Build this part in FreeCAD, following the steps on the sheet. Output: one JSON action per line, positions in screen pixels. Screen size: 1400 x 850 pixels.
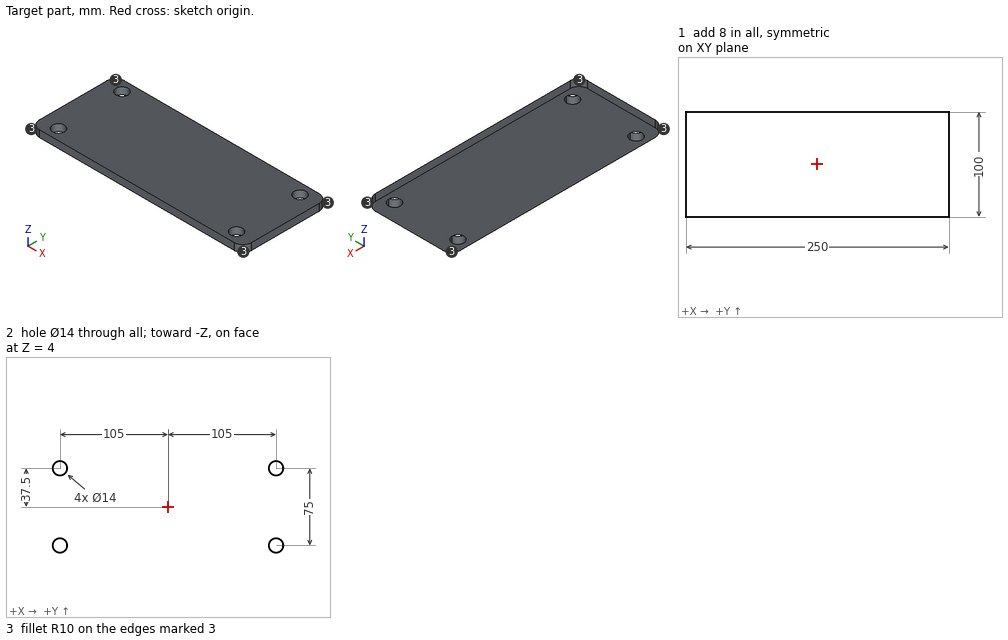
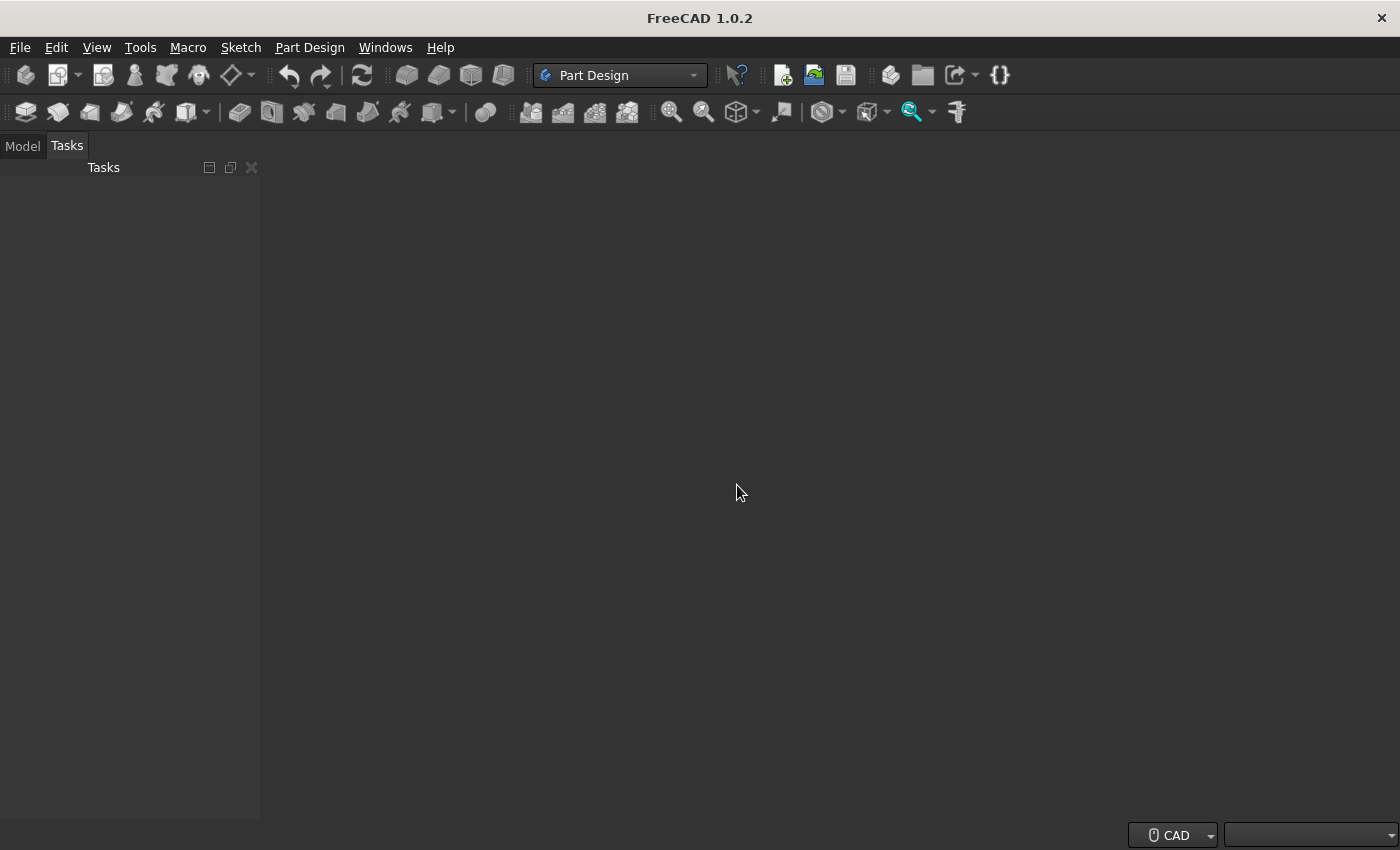
{"action": "left_click", "coordinate": [782, 76]}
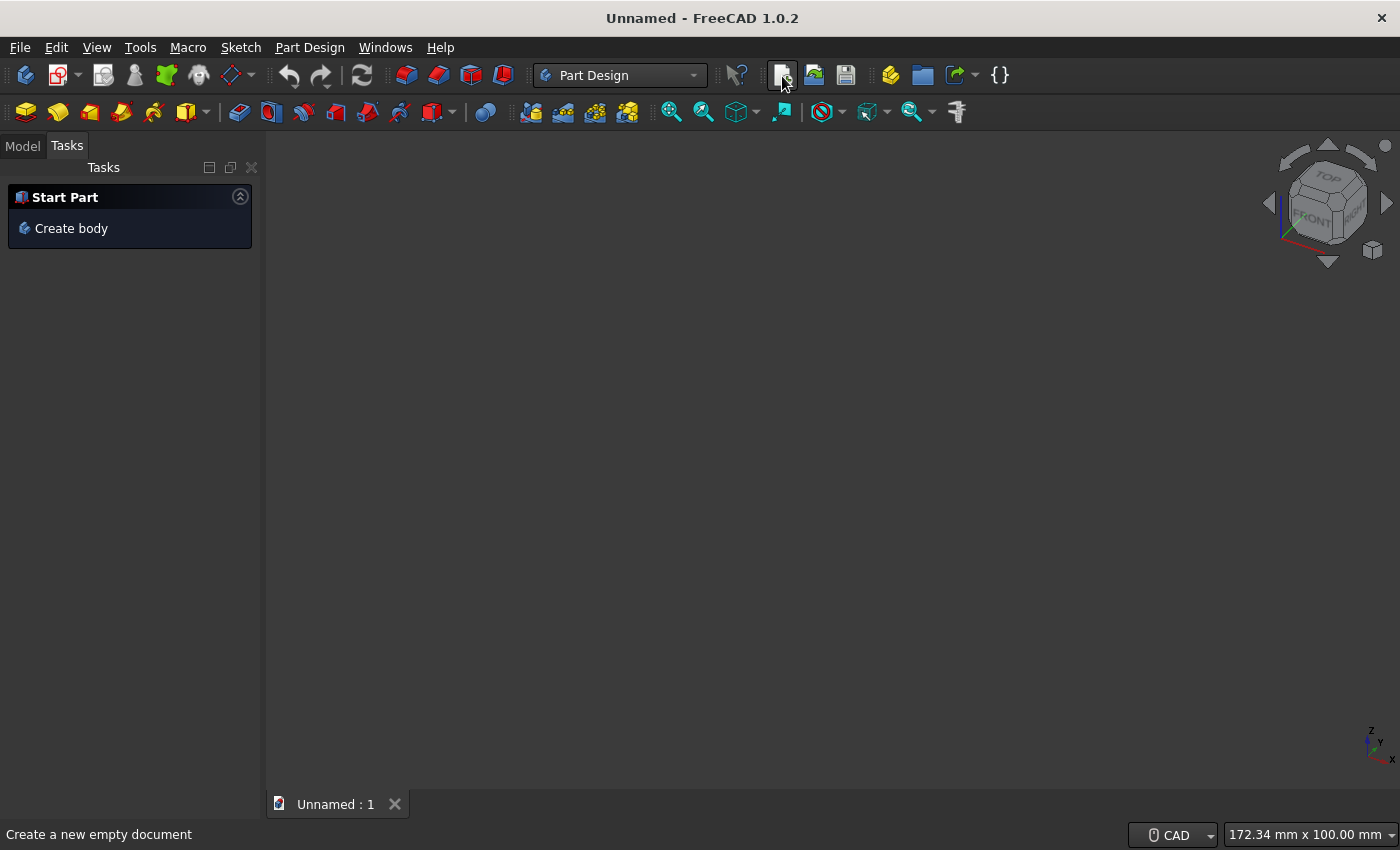
{"action": "left_click", "coordinate": [58, 76]}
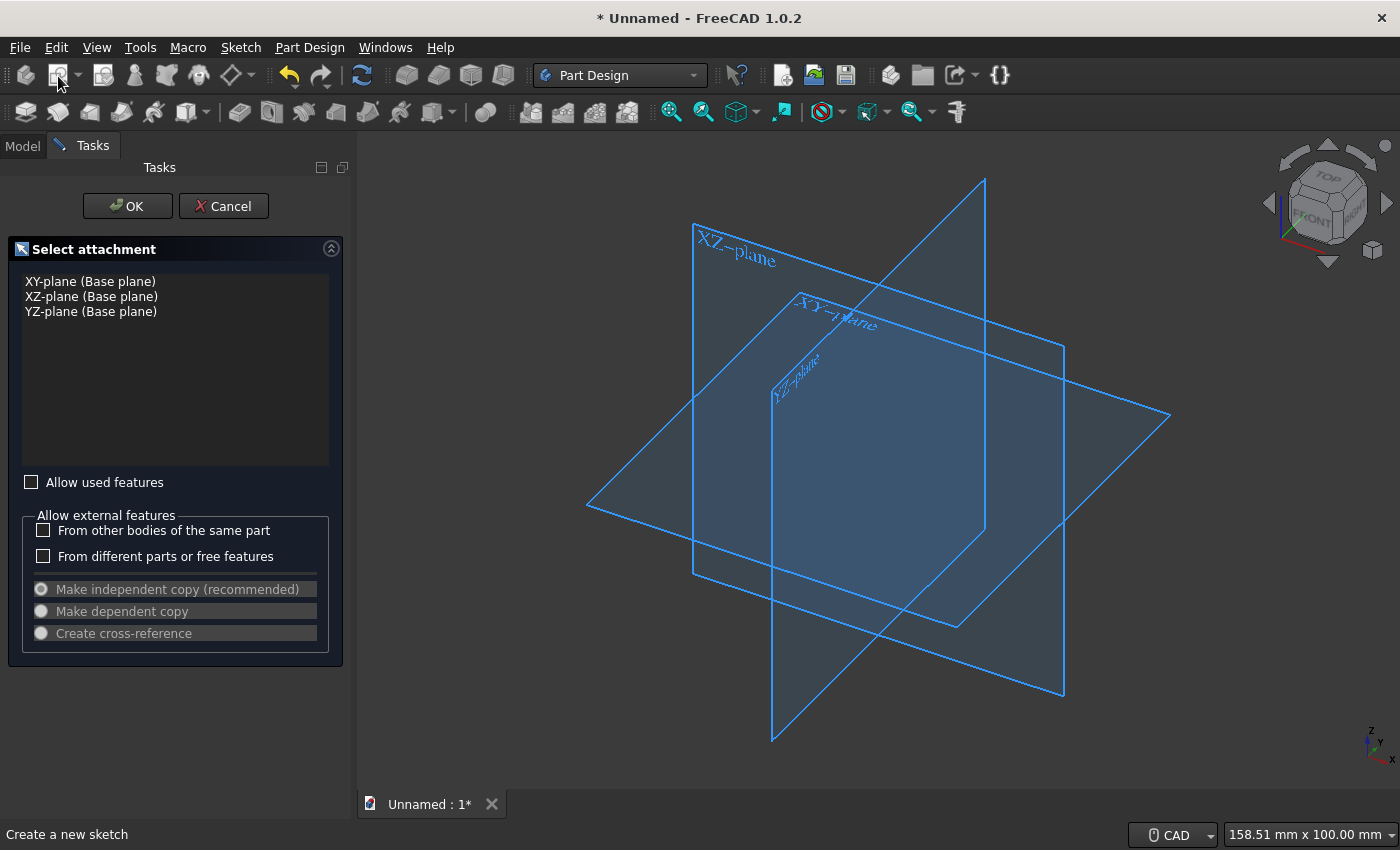
{"action": "left_click", "coordinate": [82, 282]}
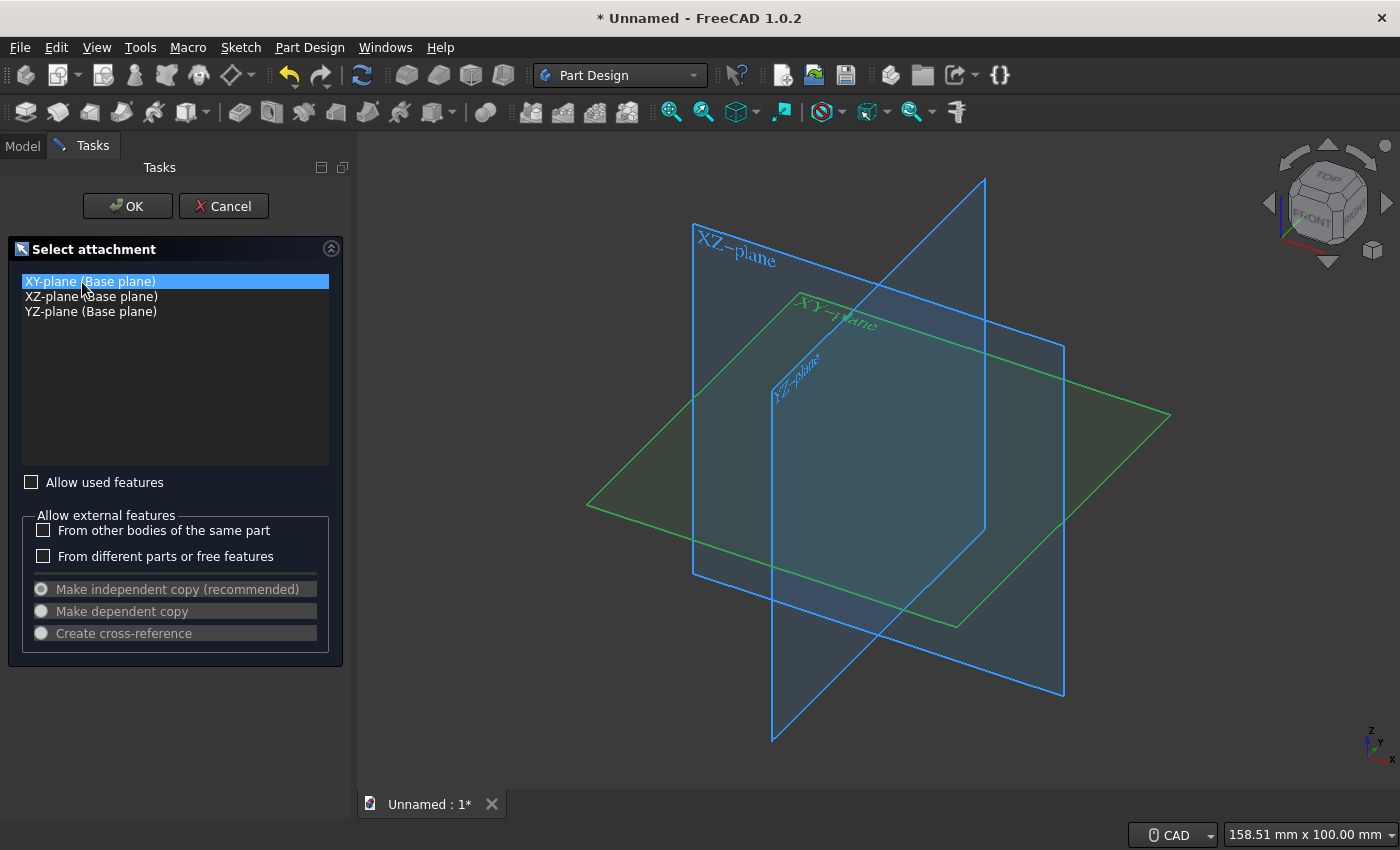
{"action": "left_click", "coordinate": [128, 206]}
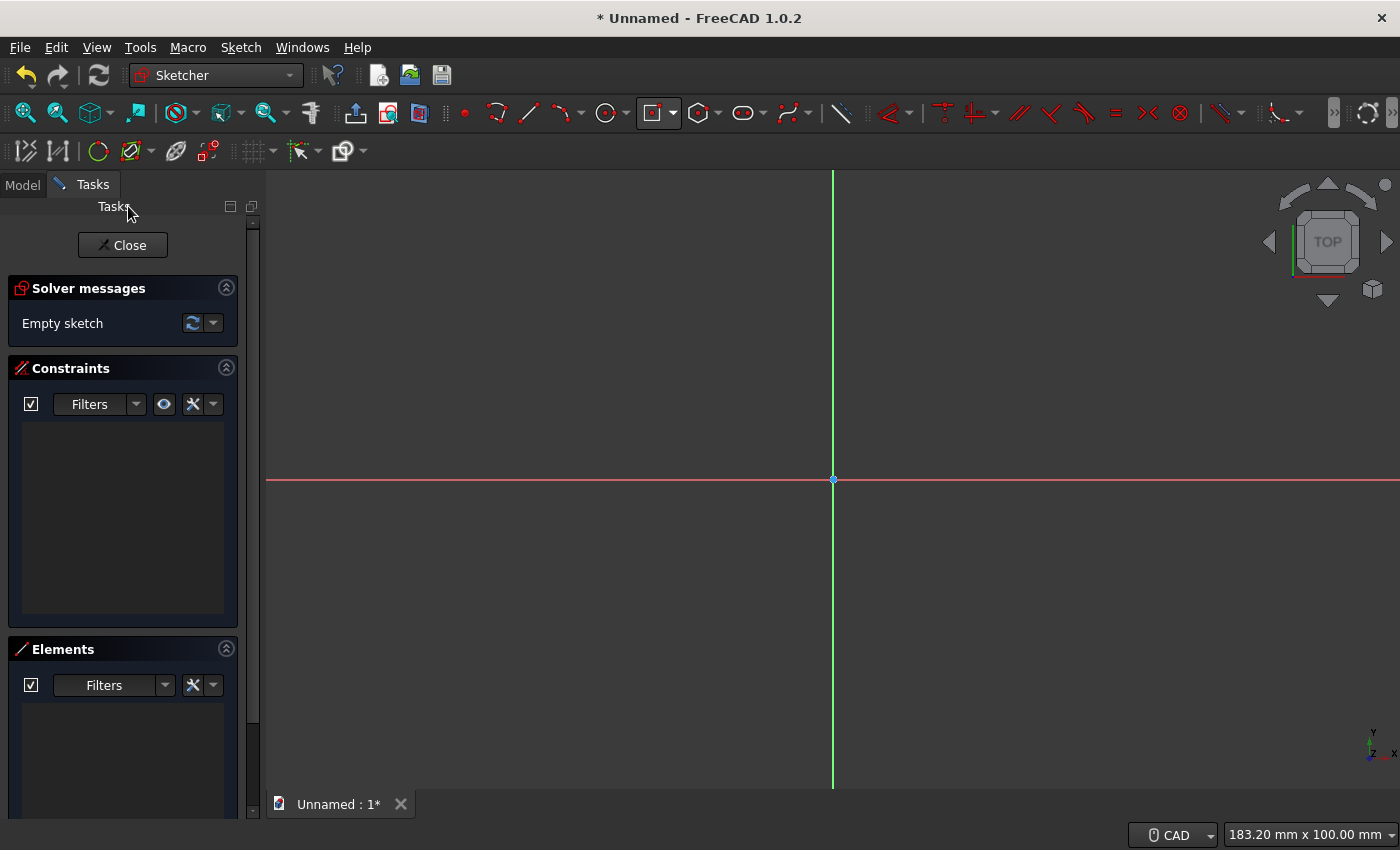
{"action": "scroll", "coordinate": [709, 480], "scroll_direction": "down", "scroll_amount": 4}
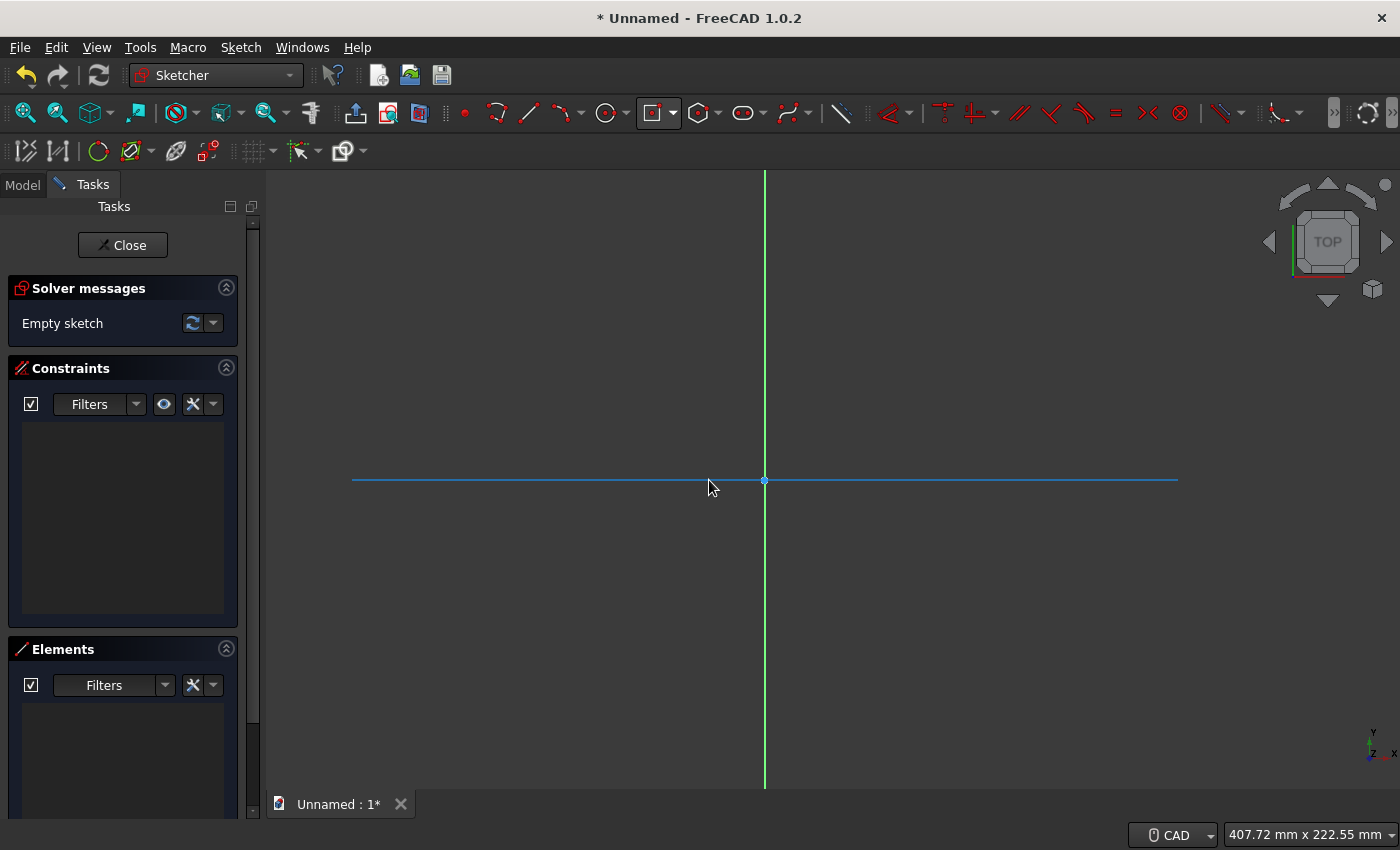
{"action": "left_click", "coordinate": [652, 114]}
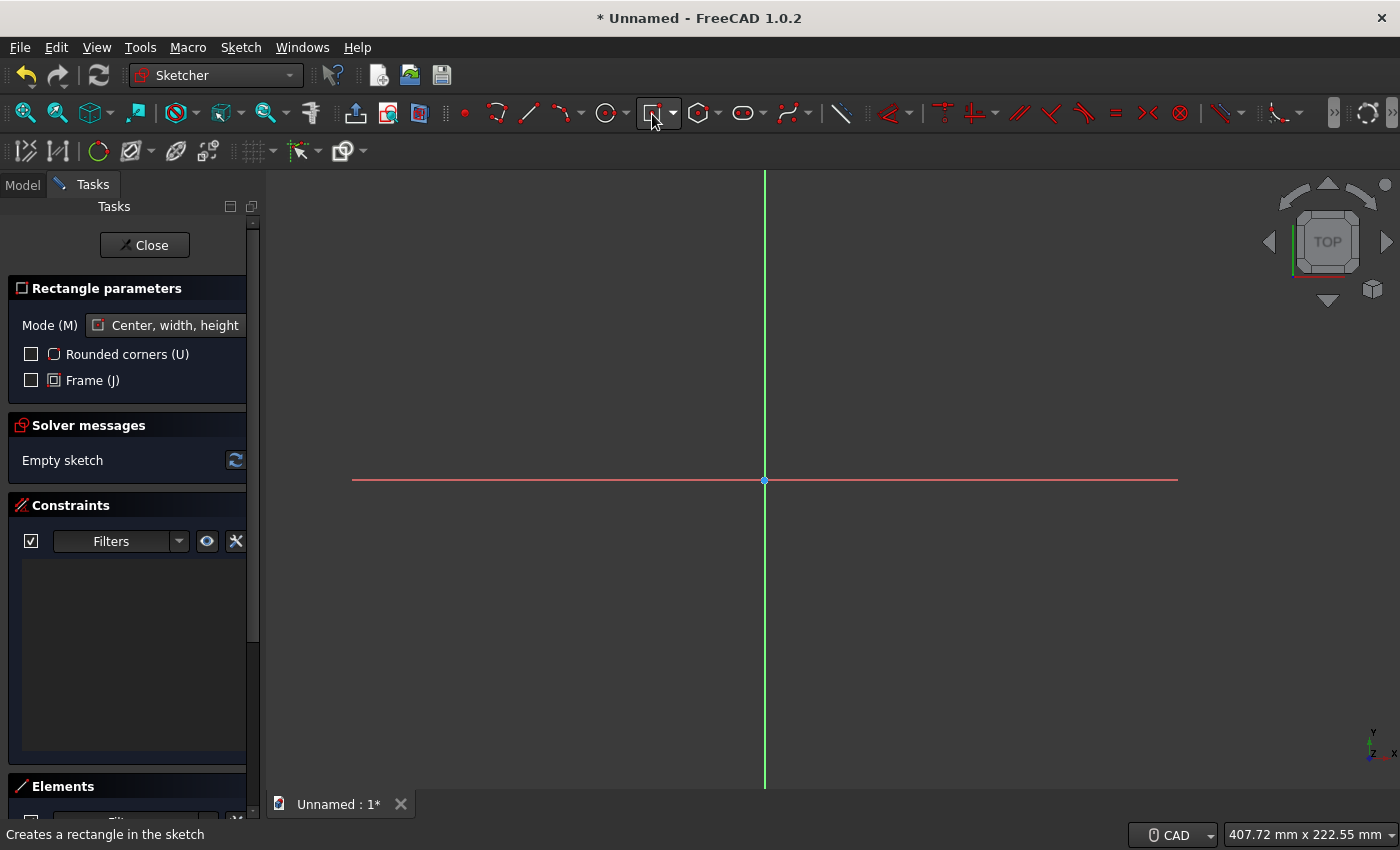
{"action": "left_click", "coordinate": [765, 480]}
{"action": "left_click", "coordinate": [1113, 341]}
{"action": "key", "text": "Escape"}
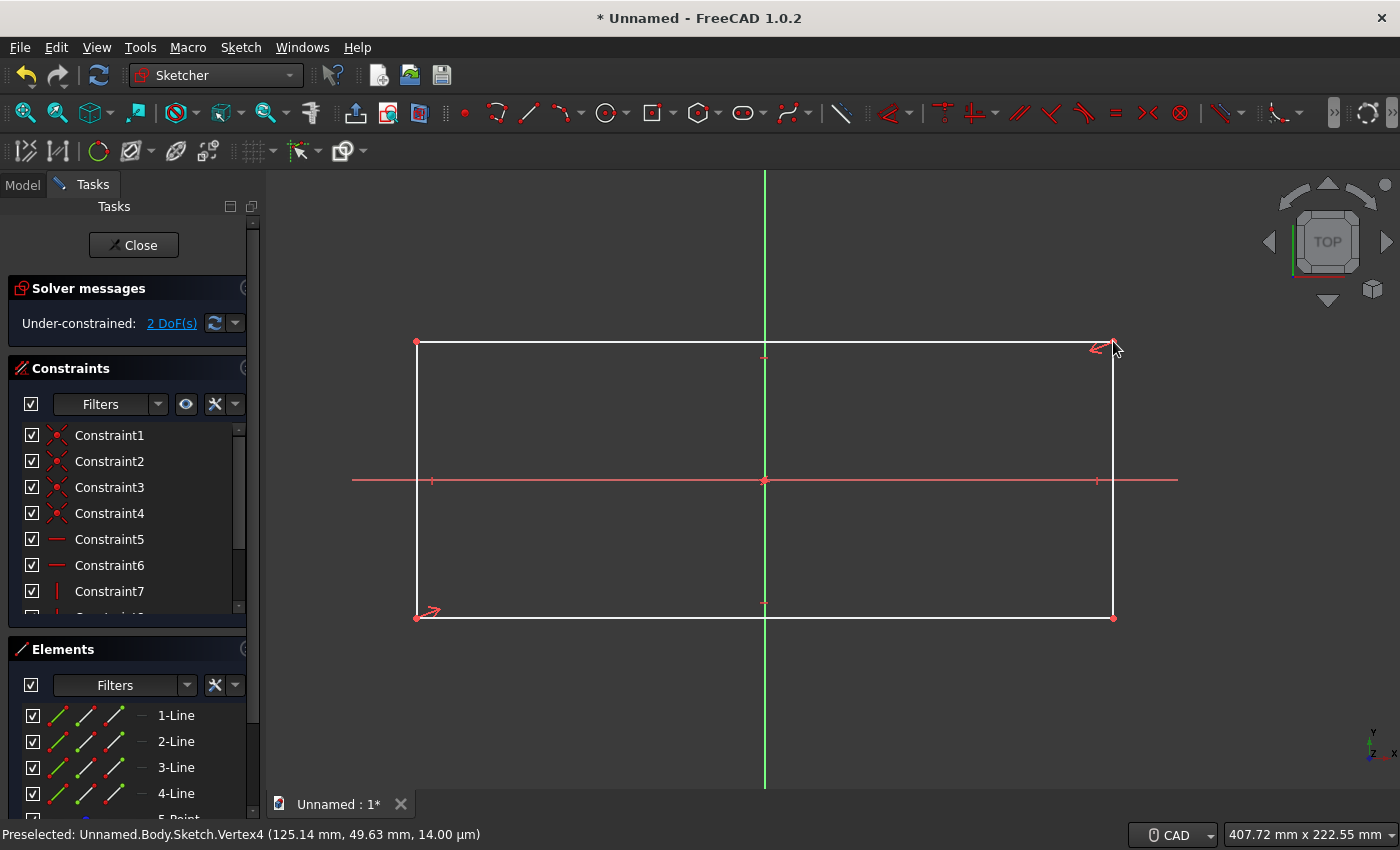
{"action": "left_click", "coordinate": [626, 618]}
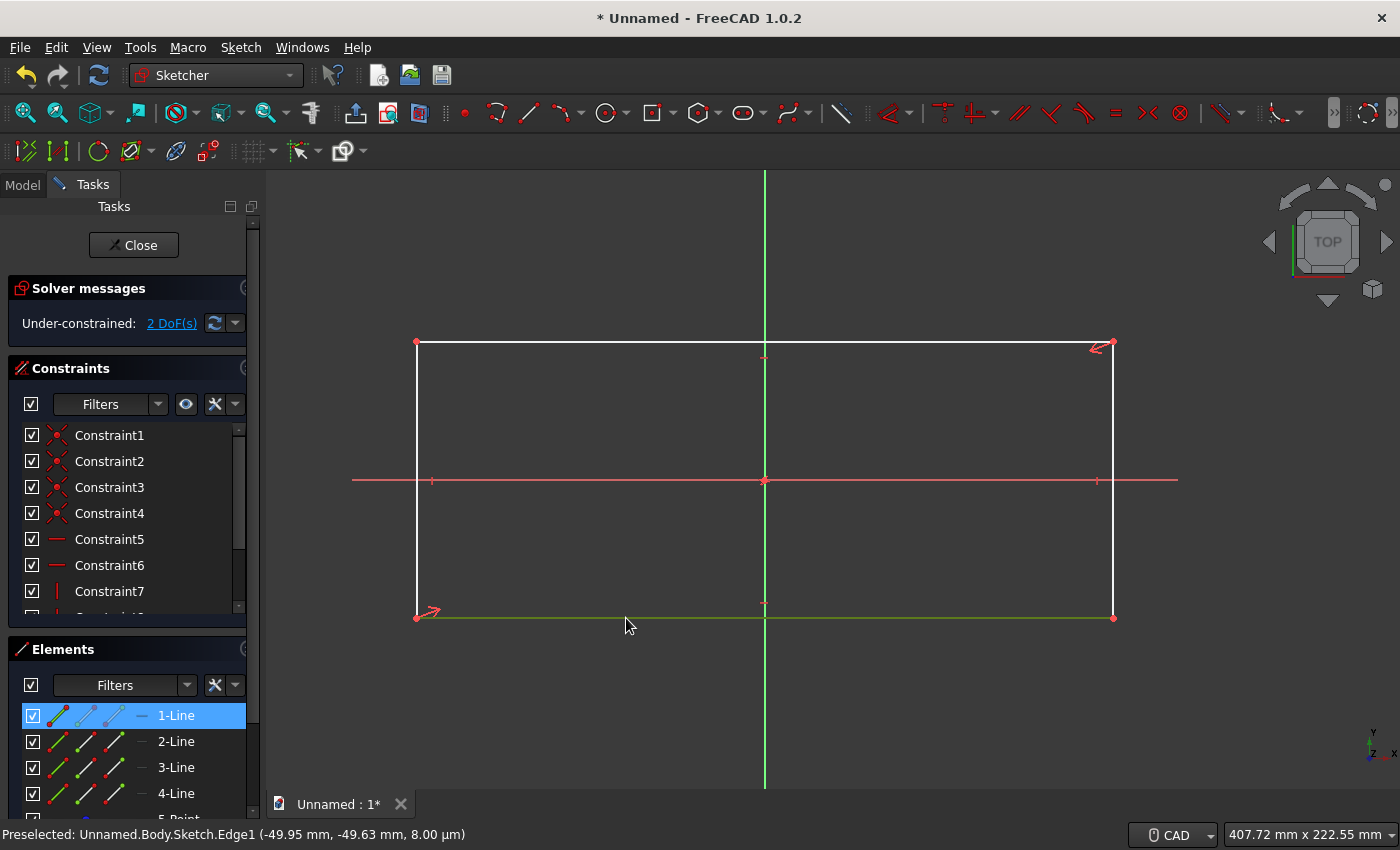
{"action": "left_click", "coordinate": [912, 114]}